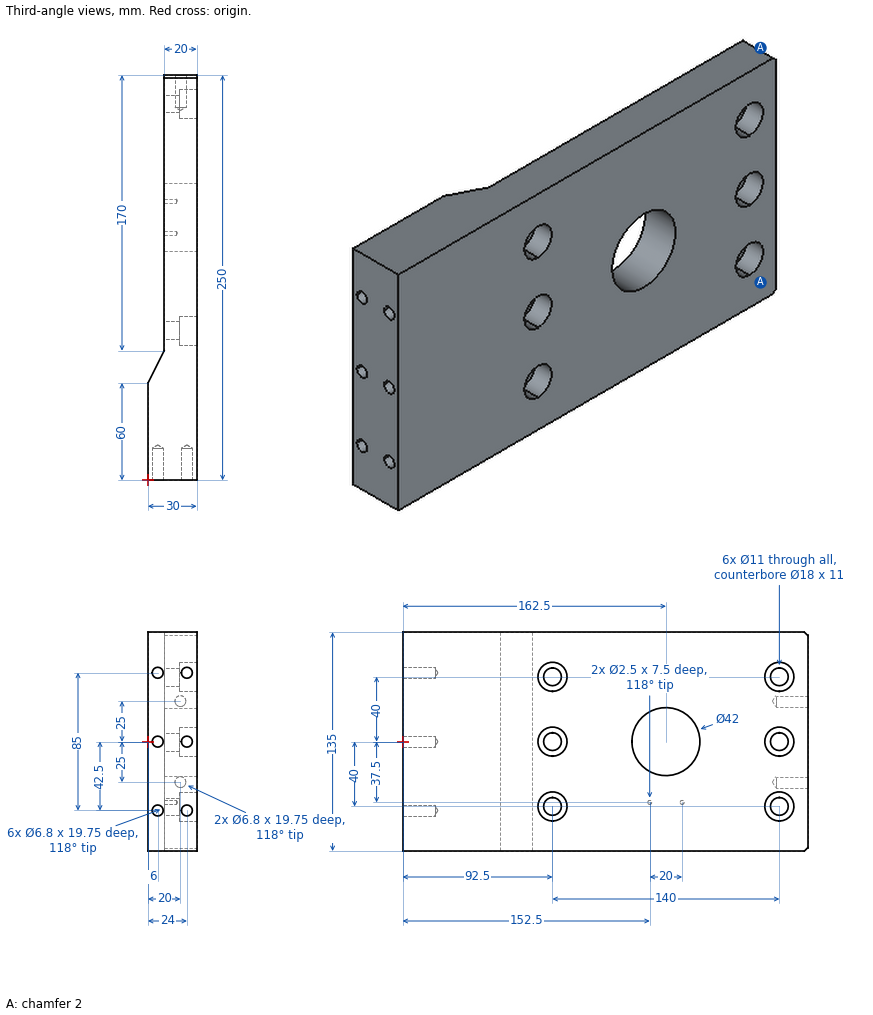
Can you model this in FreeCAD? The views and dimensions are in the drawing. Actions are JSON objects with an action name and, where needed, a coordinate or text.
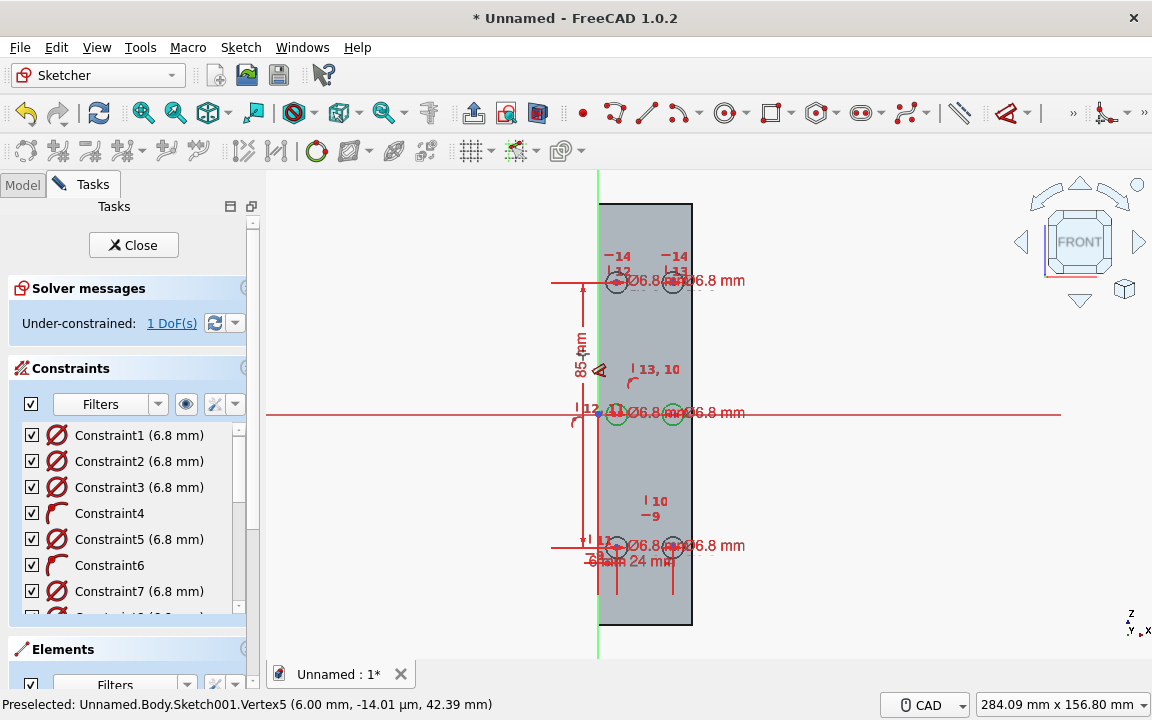
{"action": "left_click", "coordinate": [617, 548]}
{"action": "left_click", "coordinate": [564, 481]}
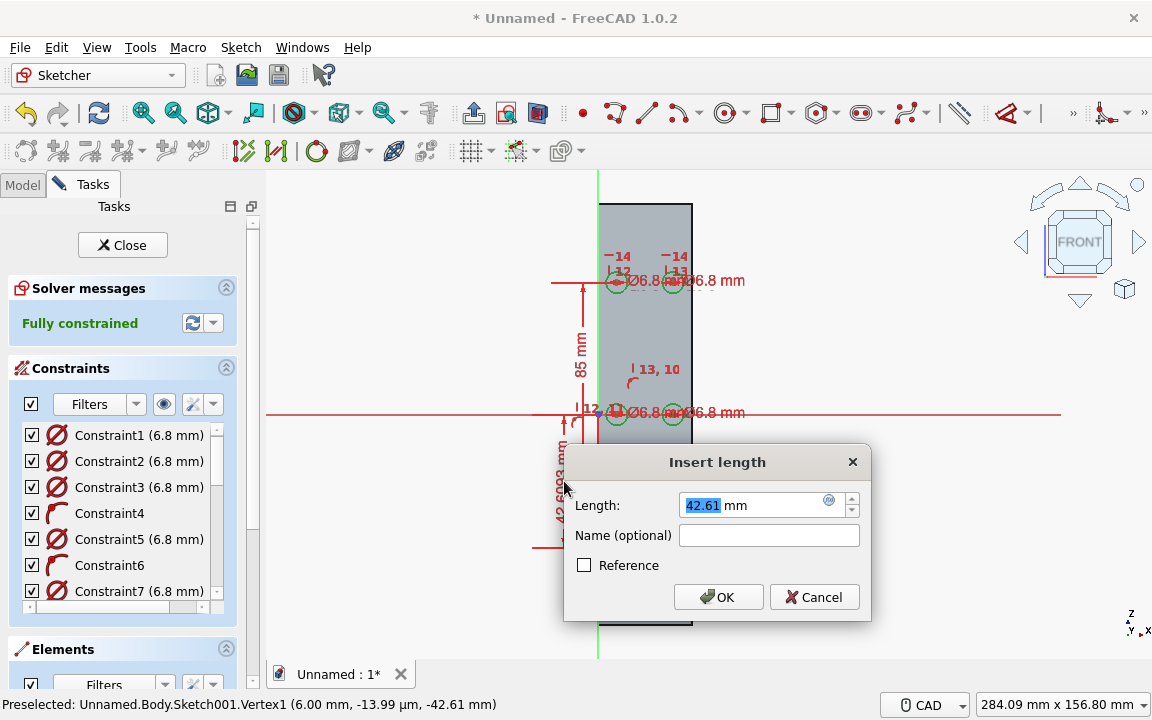
{"action": "type", "text": "42.5"}
{"action": "key", "text": "Return"}
{"action": "key", "text": "Escape"}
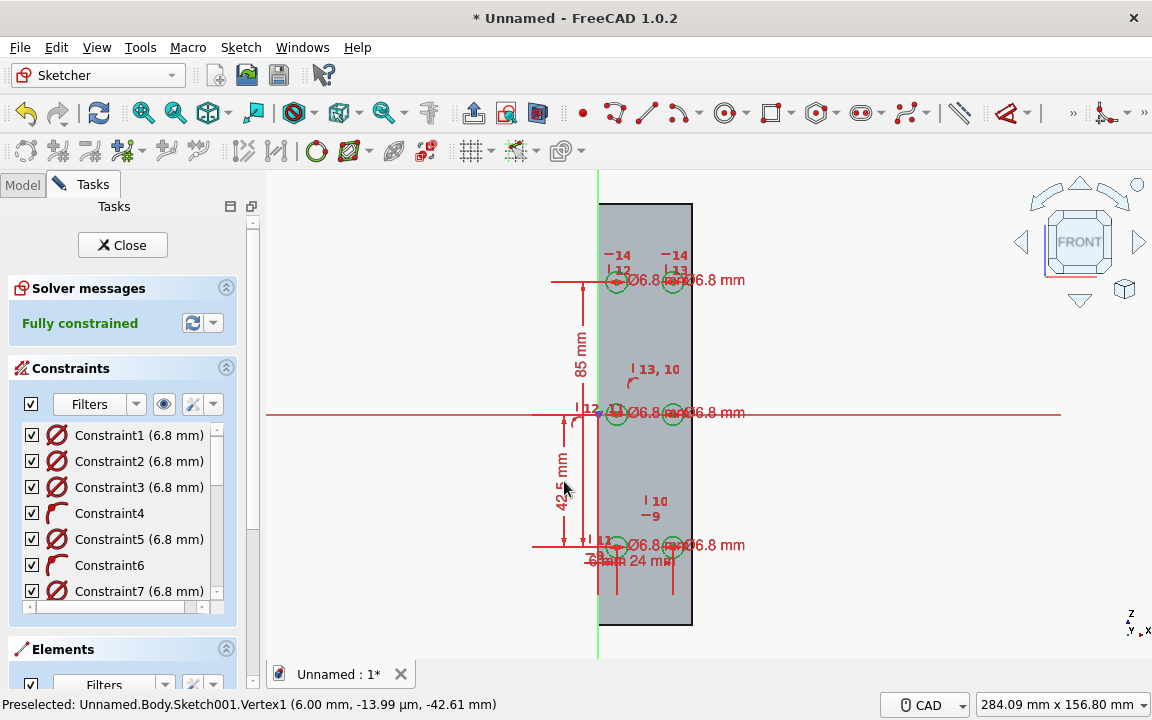
{"action": "left_click", "coordinate": [123, 245]}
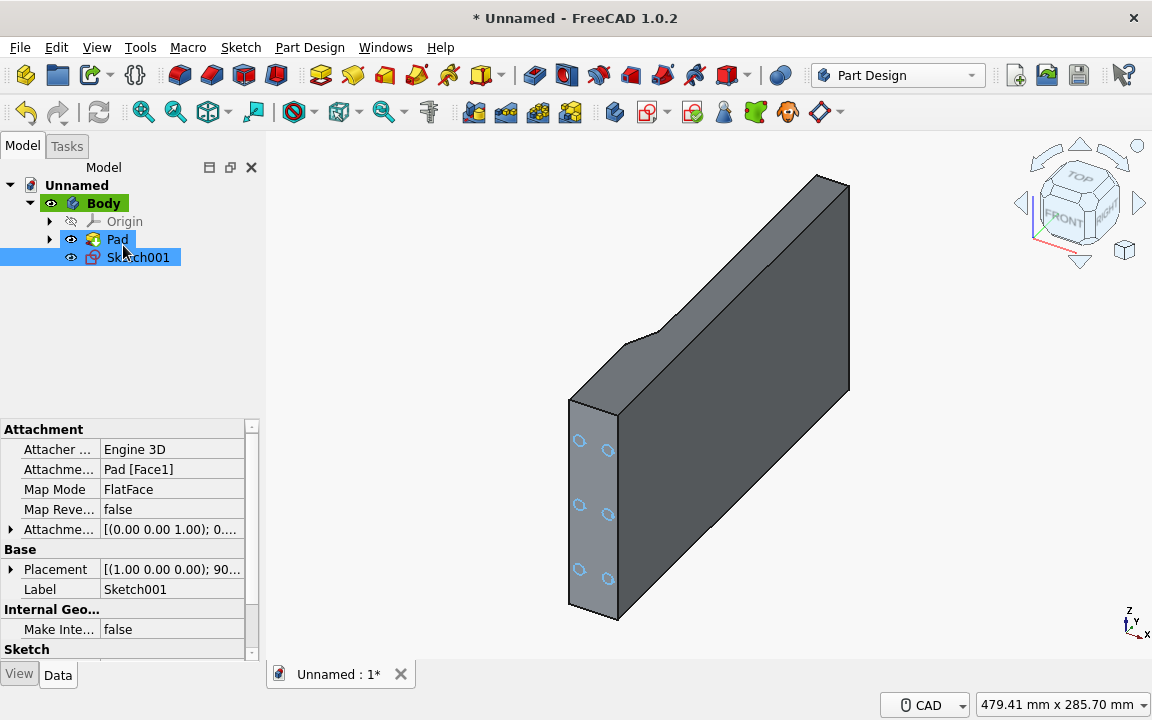
{"action": "left_click", "coordinate": [568, 76]}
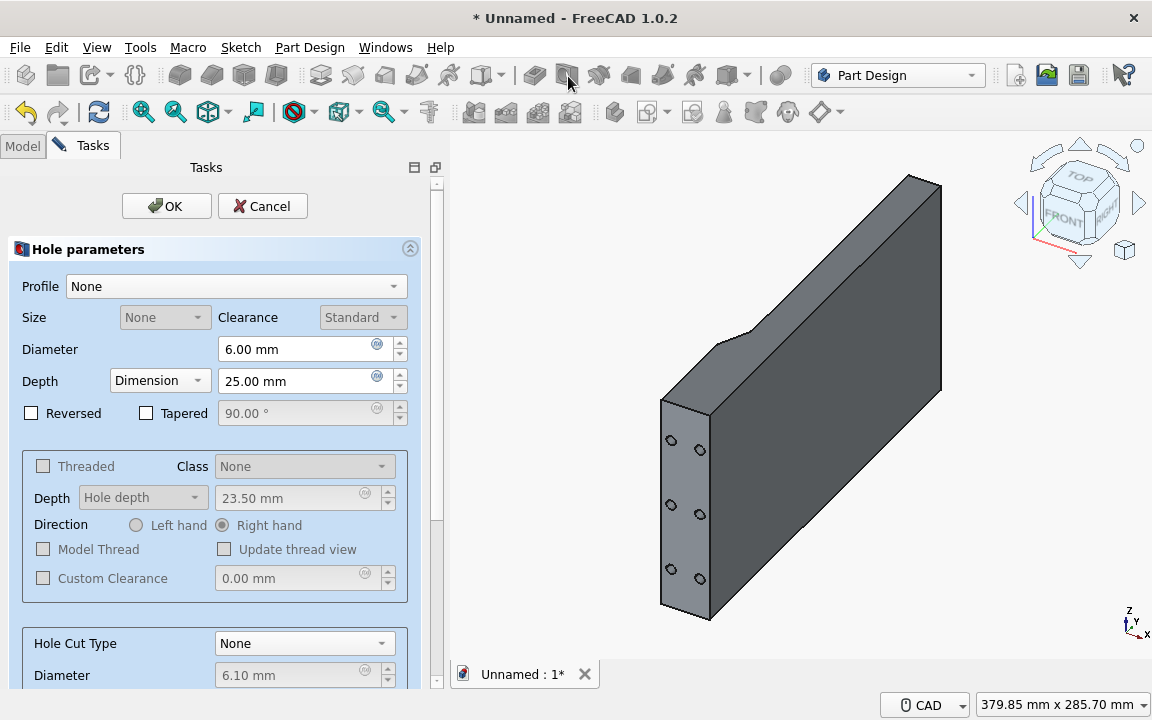
{"action": "triple_click", "coordinate": [305, 349]}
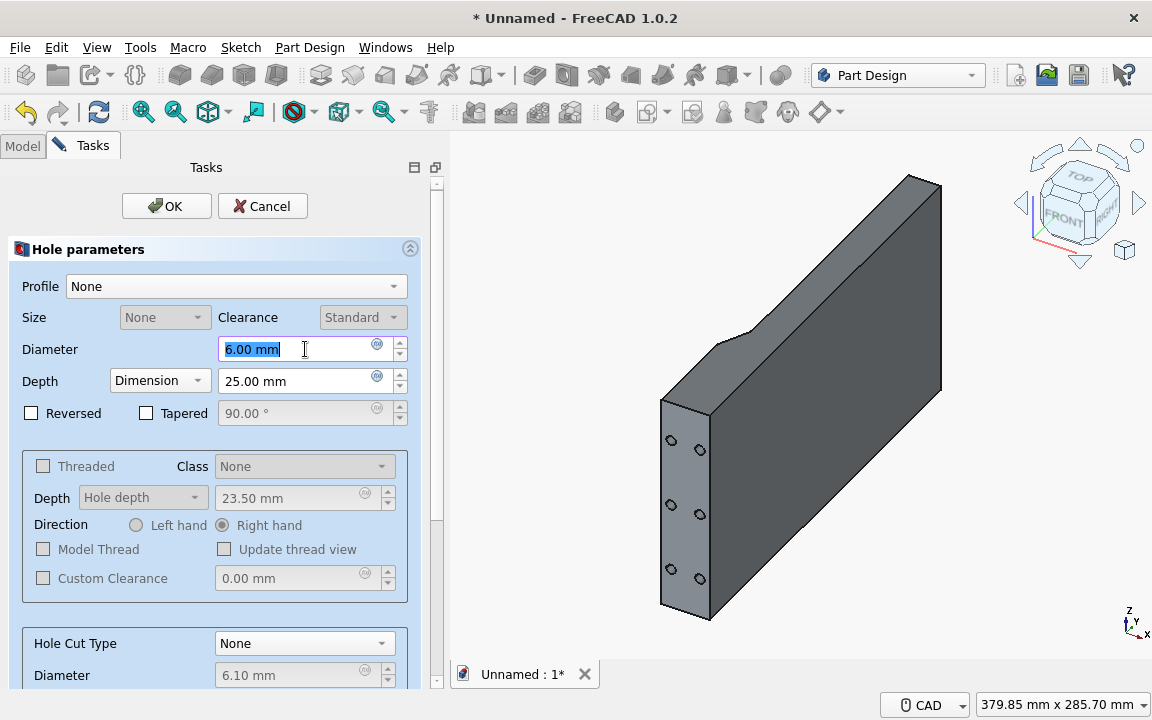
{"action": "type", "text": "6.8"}
{"action": "key", "text": "Tab"}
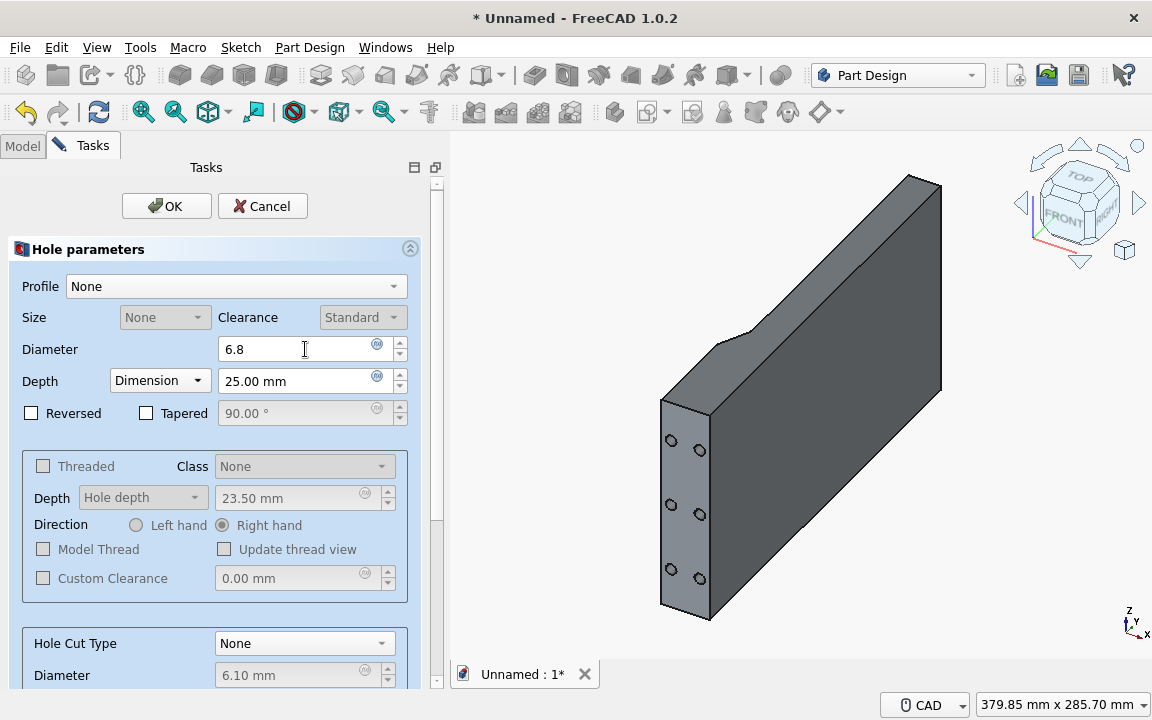
{"action": "triple_click", "coordinate": [305, 381]}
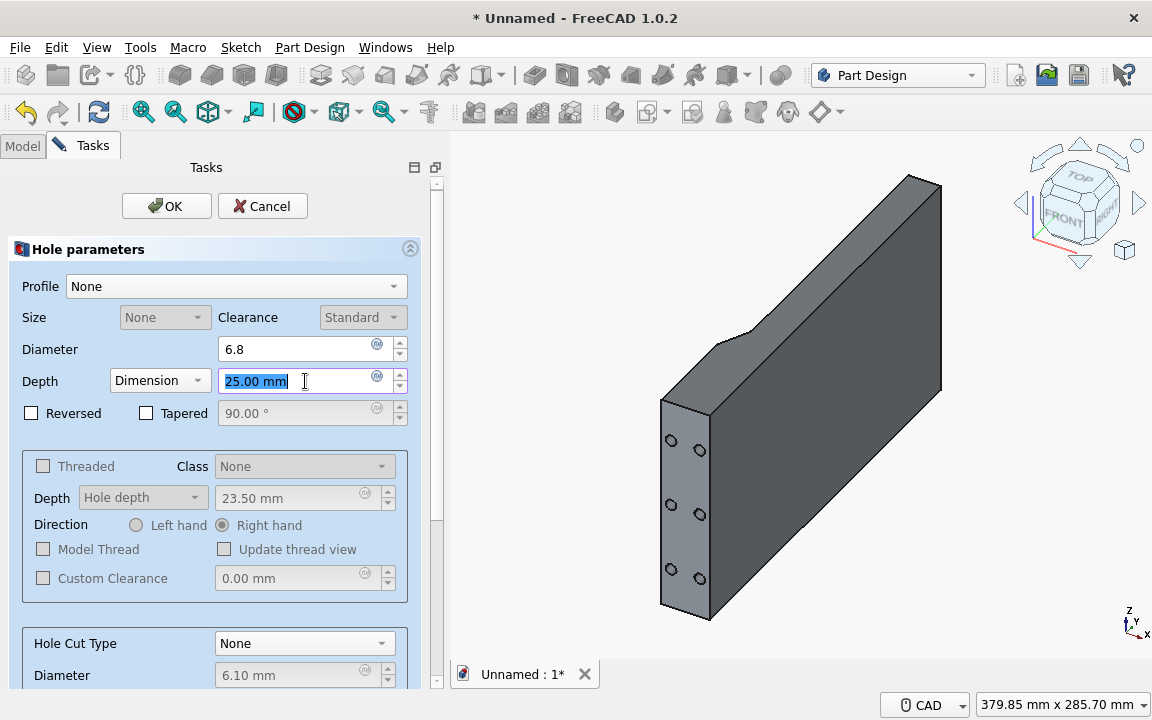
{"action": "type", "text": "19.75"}
{"action": "key", "text": "Tab"}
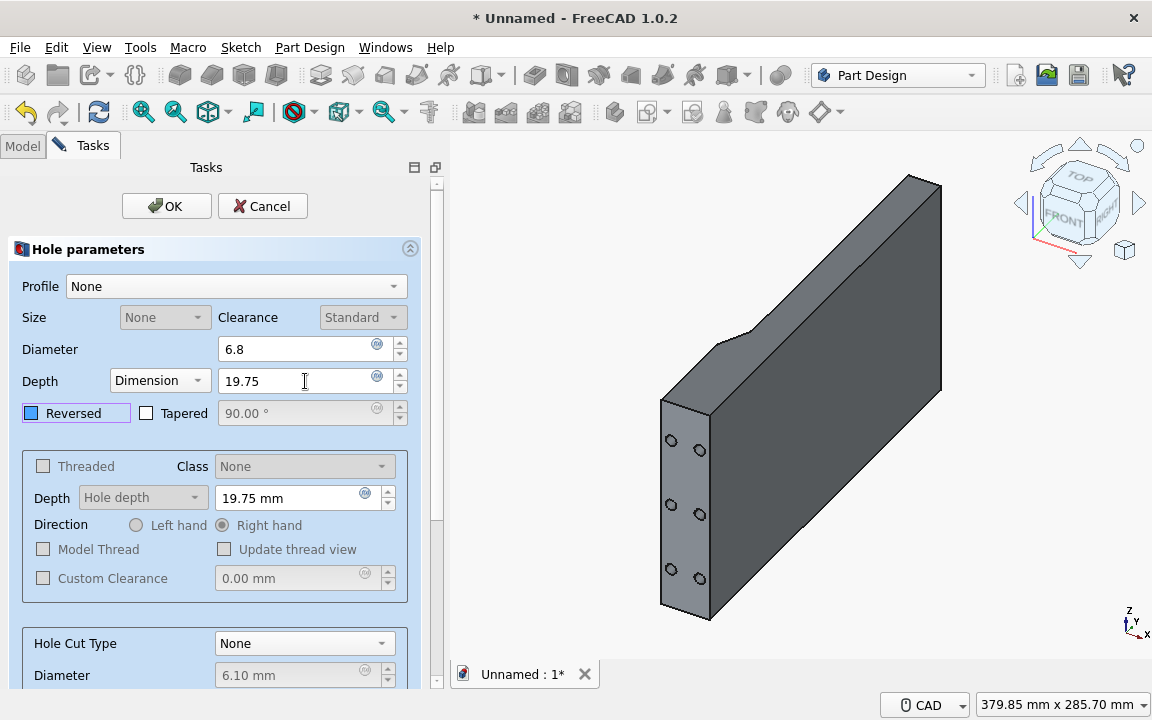
{"action": "left_click", "coordinate": [167, 206]}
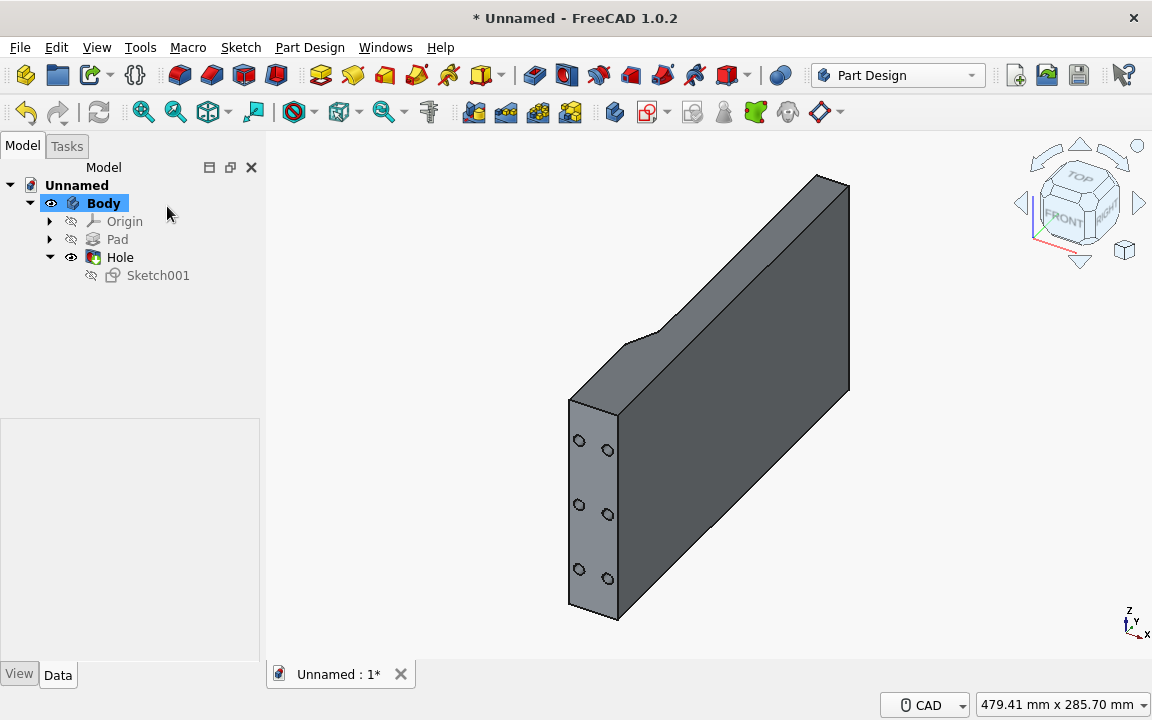
{"action": "left_click", "coordinate": [766, 369]}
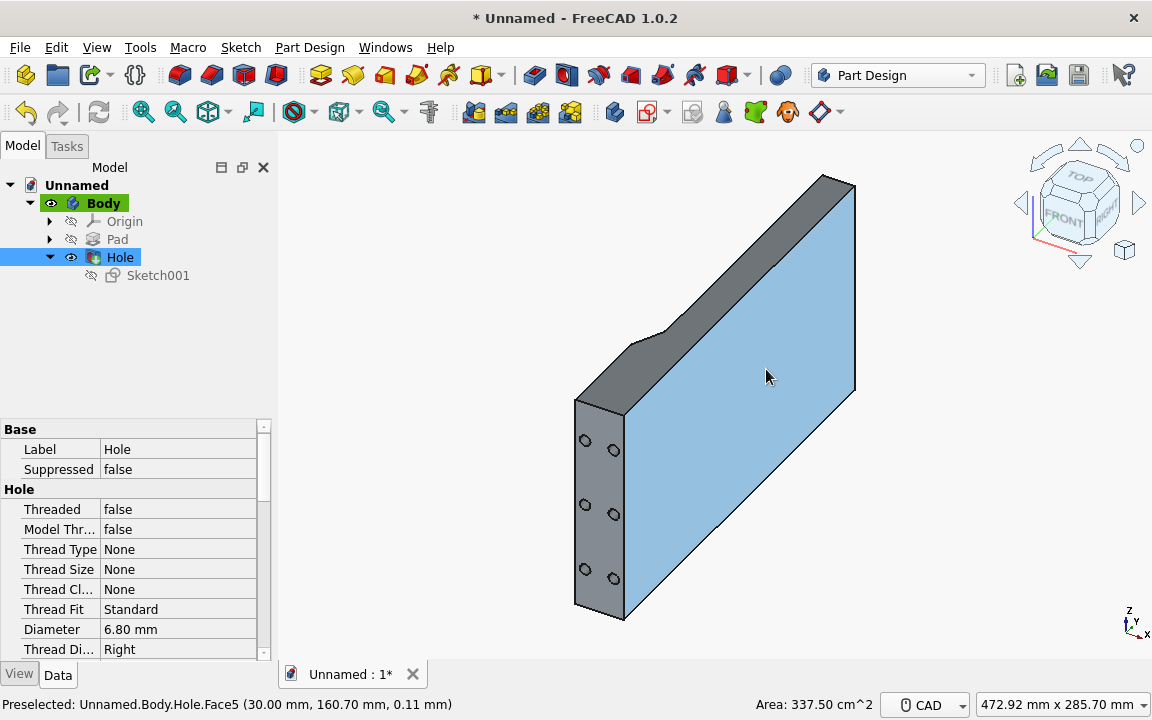
{"action": "left_click", "coordinate": [648, 112]}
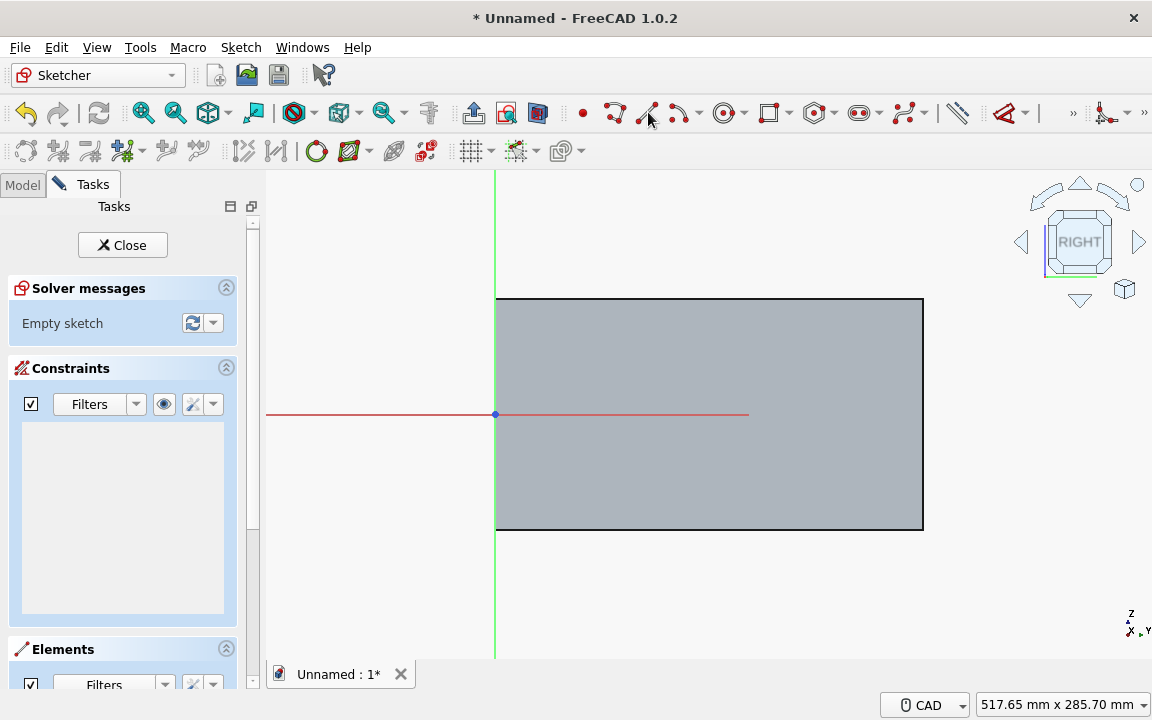
{"action": "left_click", "coordinate": [724, 114]}